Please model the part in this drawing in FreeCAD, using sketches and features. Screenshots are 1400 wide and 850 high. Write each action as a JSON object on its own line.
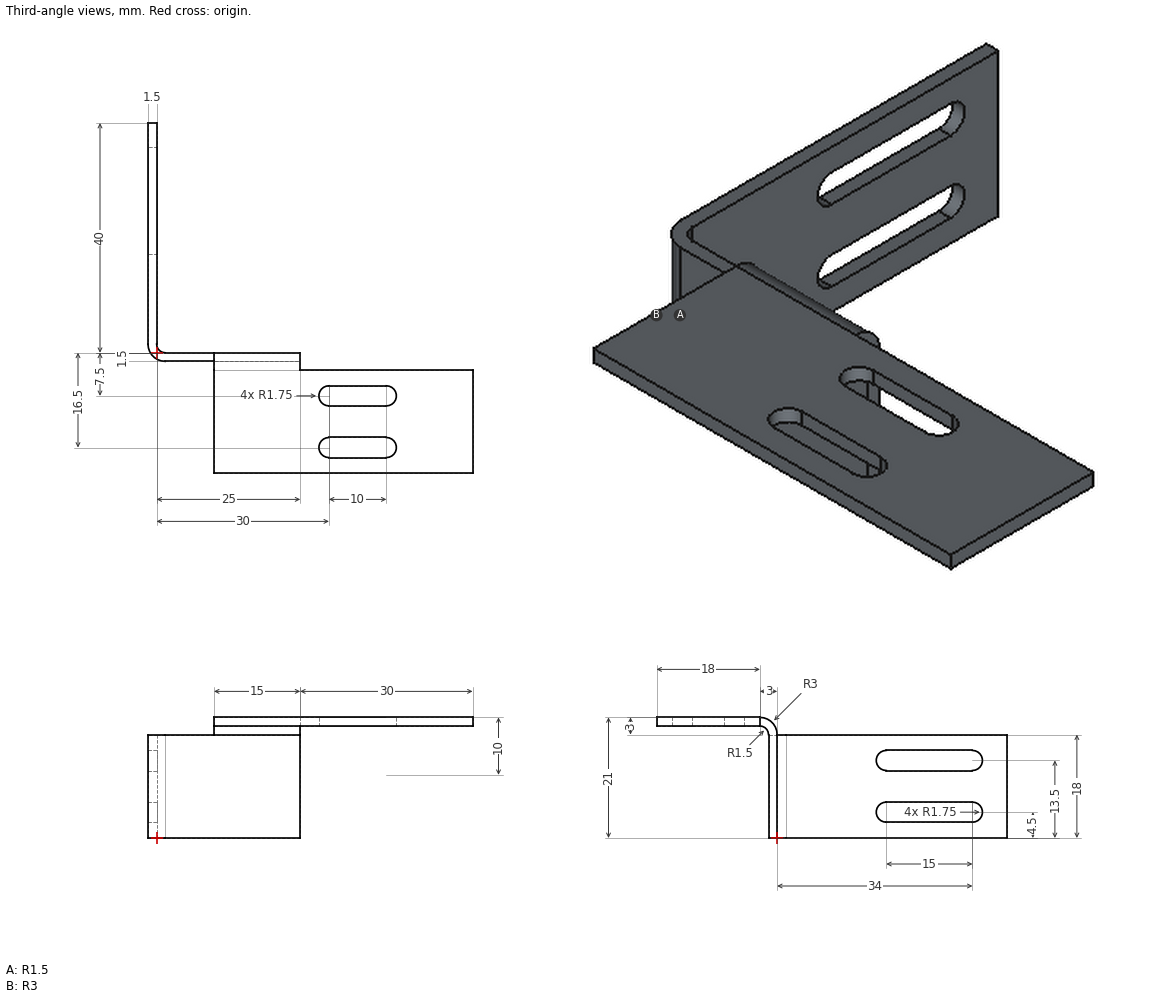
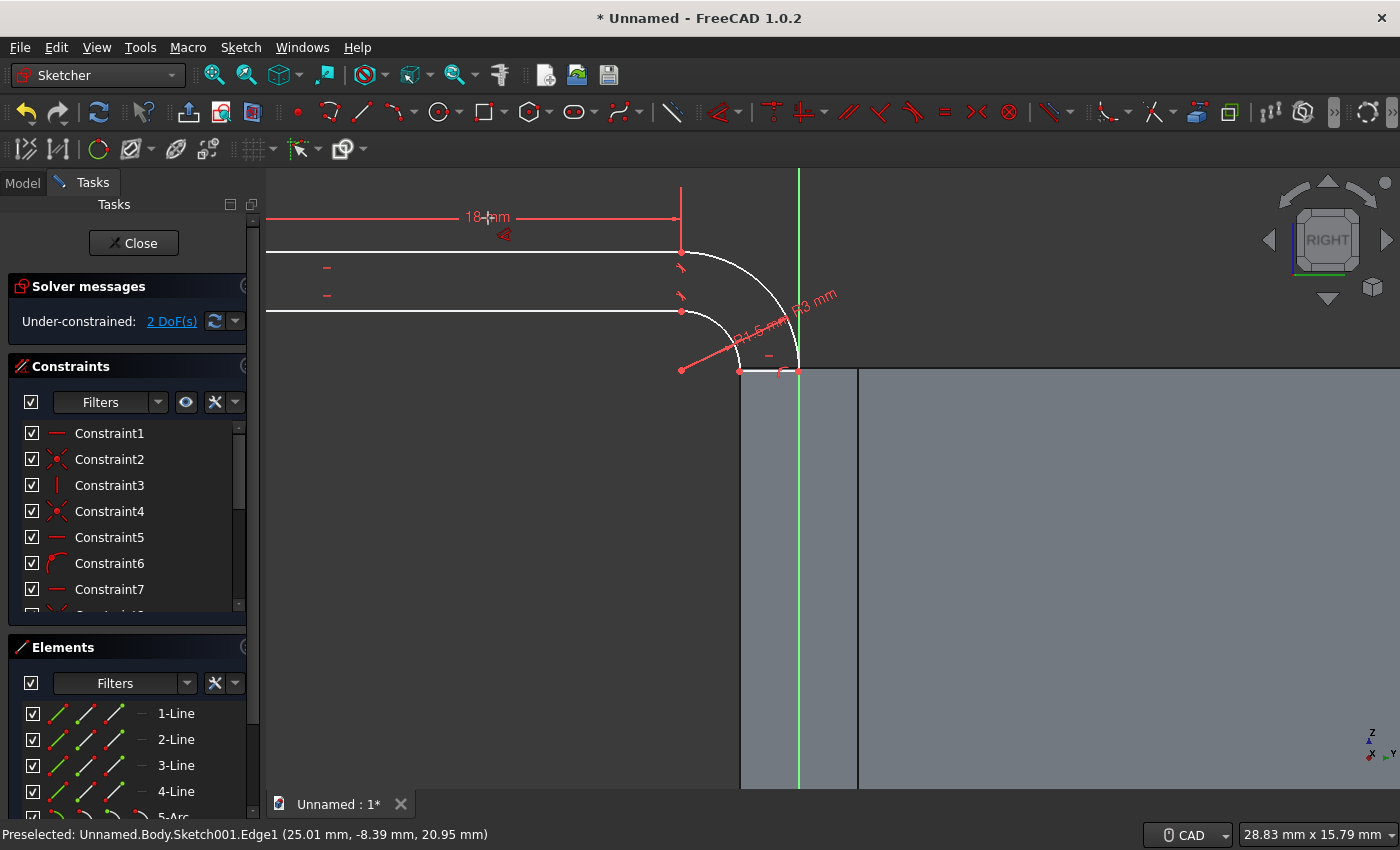
{"action": "left_click", "coordinate": [681, 252]}
{"action": "left_click", "coordinate": [833, 507]}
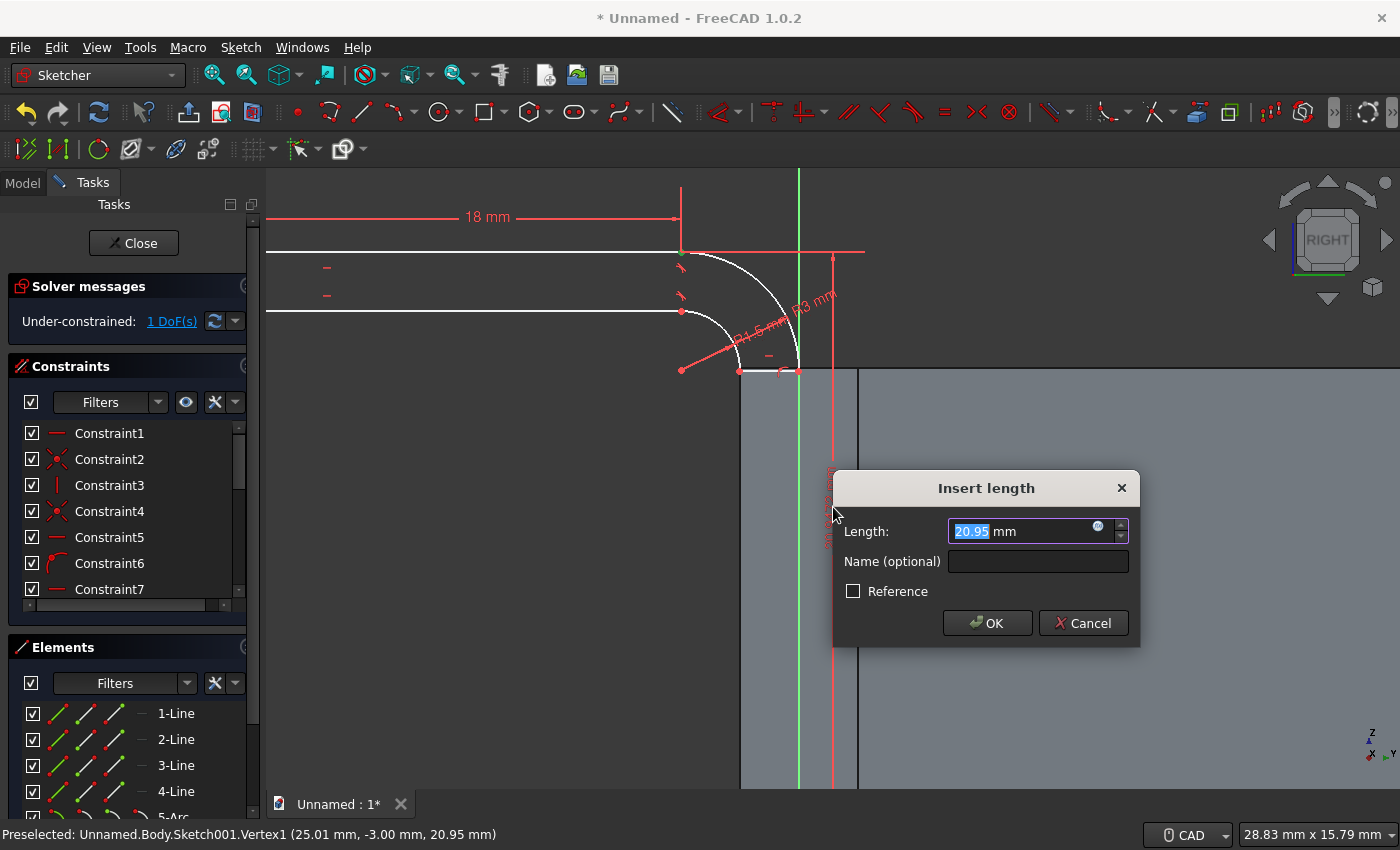
{"action": "type", "text": "21"}
{"action": "key", "text": "Return"}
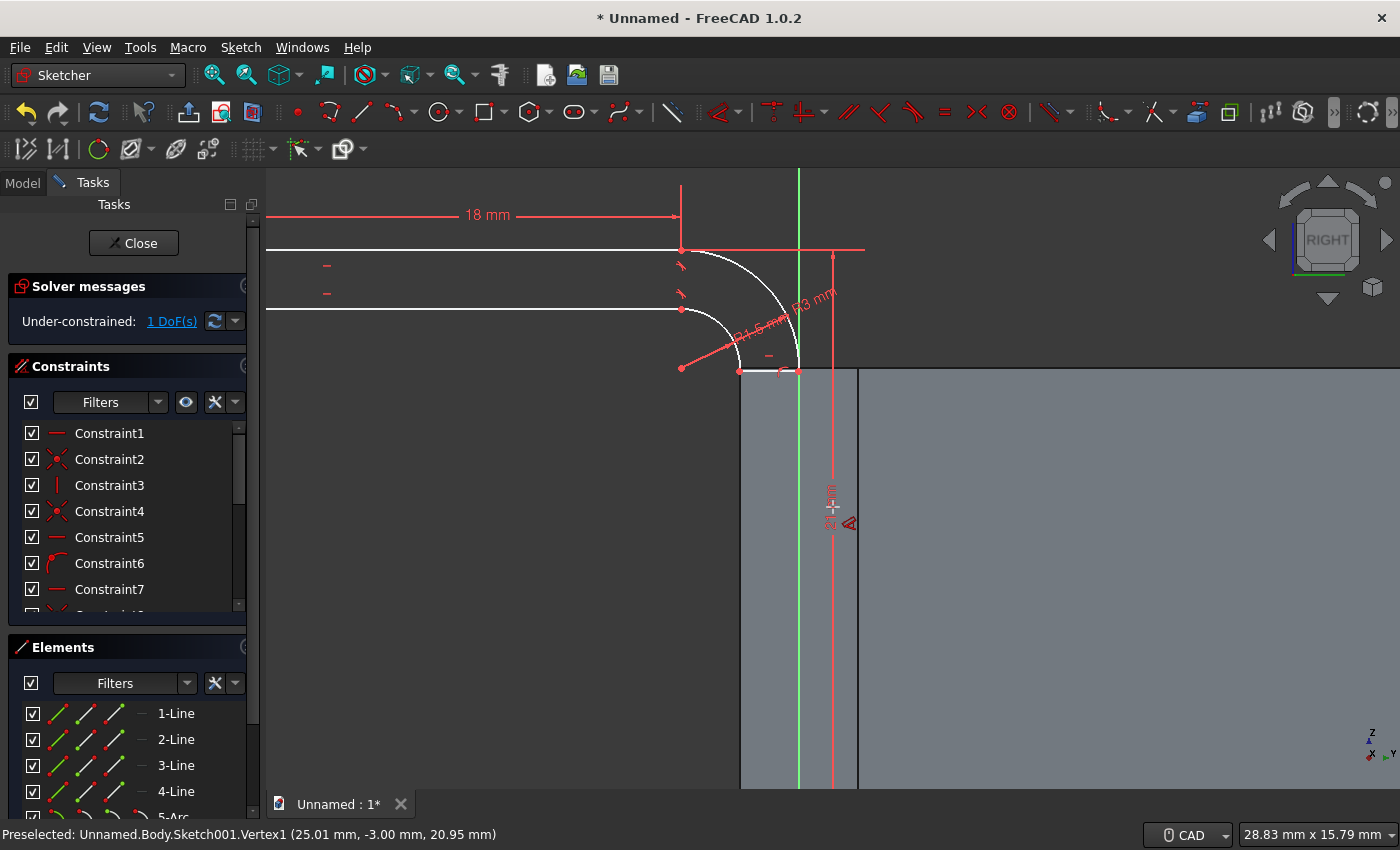
{"action": "left_click", "coordinate": [740, 371]}
{"action": "left_click", "coordinate": [833, 566]}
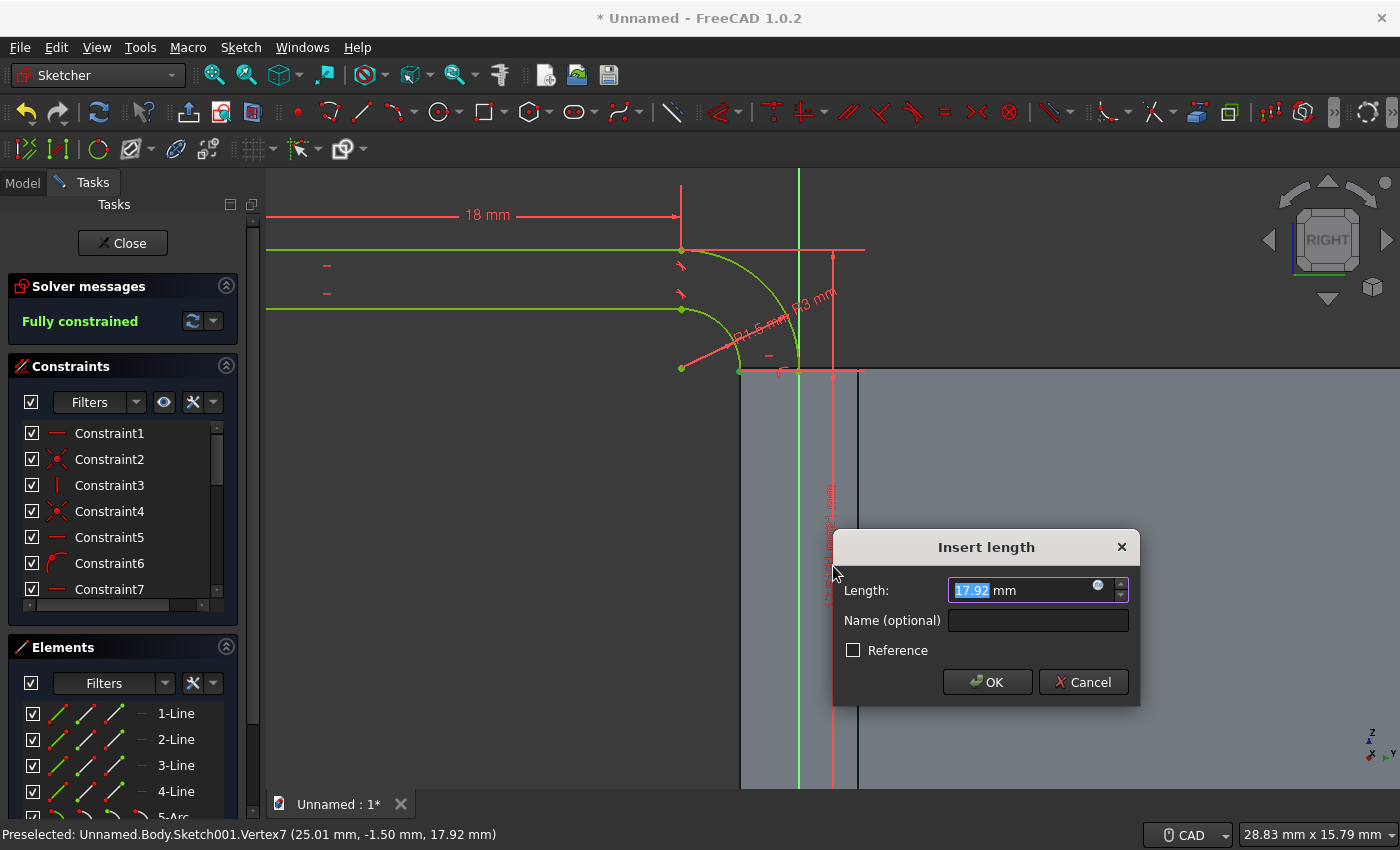
{"action": "type", "text": "18"}
{"action": "key", "text": "Return"}
{"action": "key", "text": "Escape"}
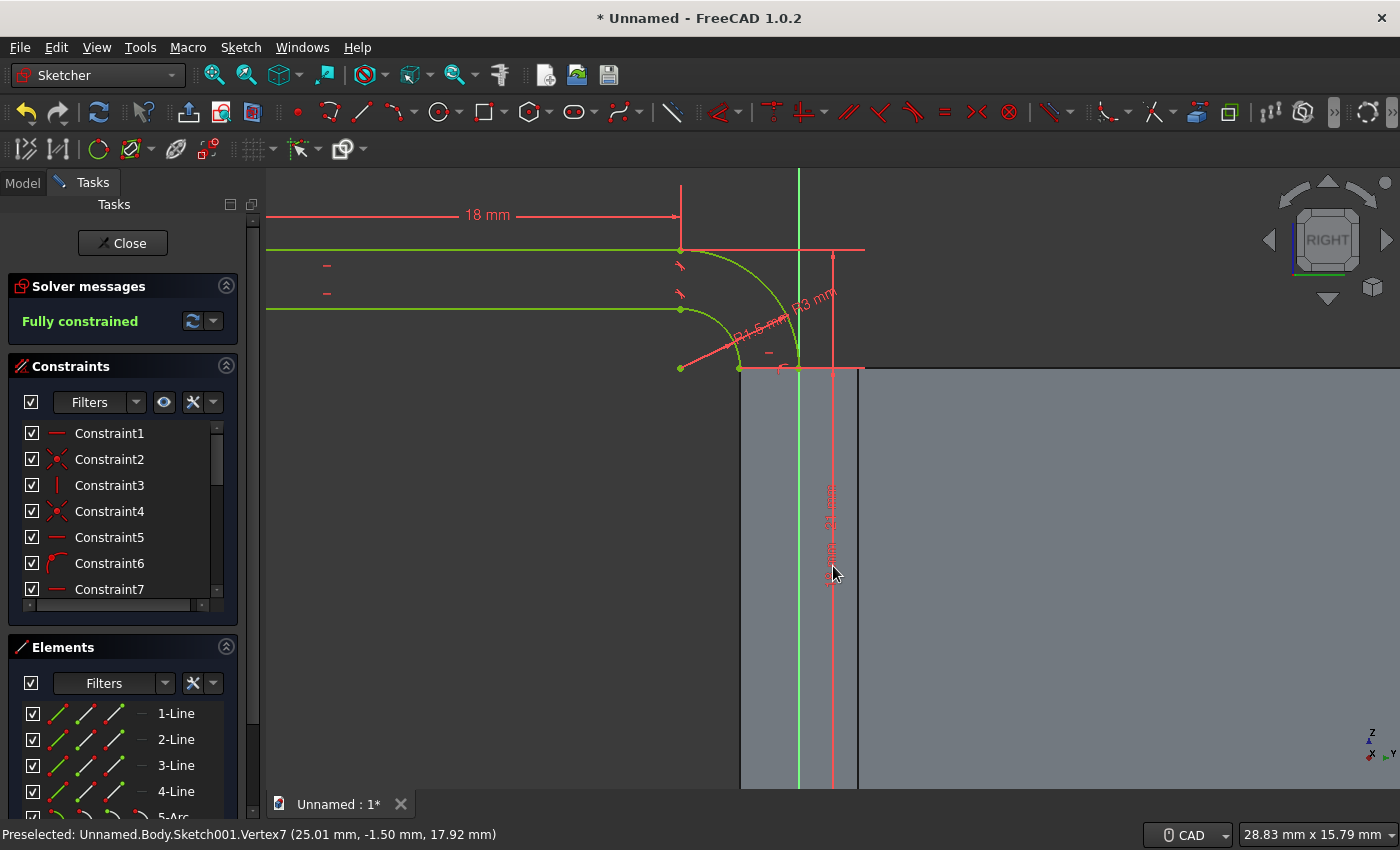
{"action": "left_click", "coordinate": [123, 243]}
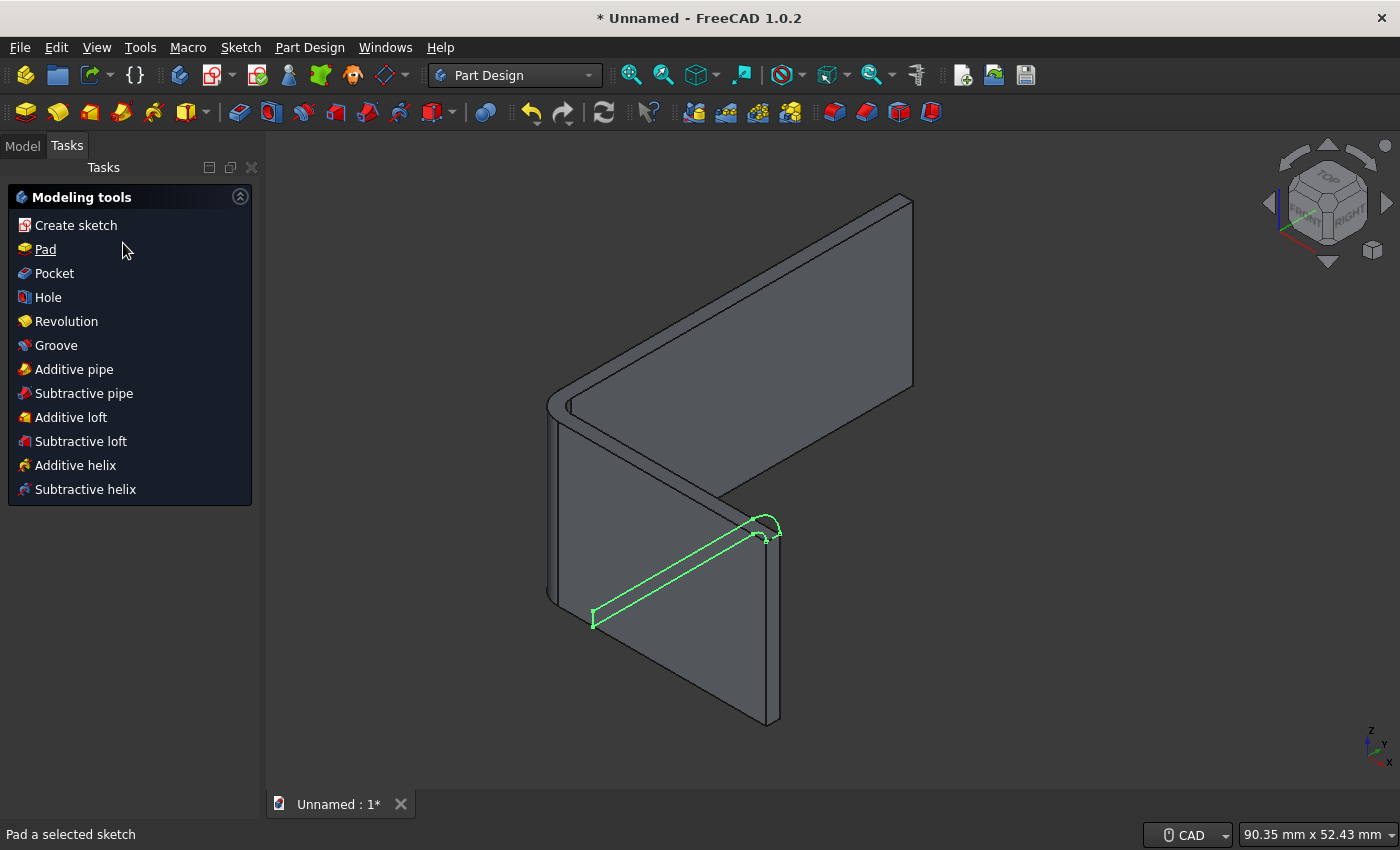
{"action": "left_click", "coordinate": [26, 112]}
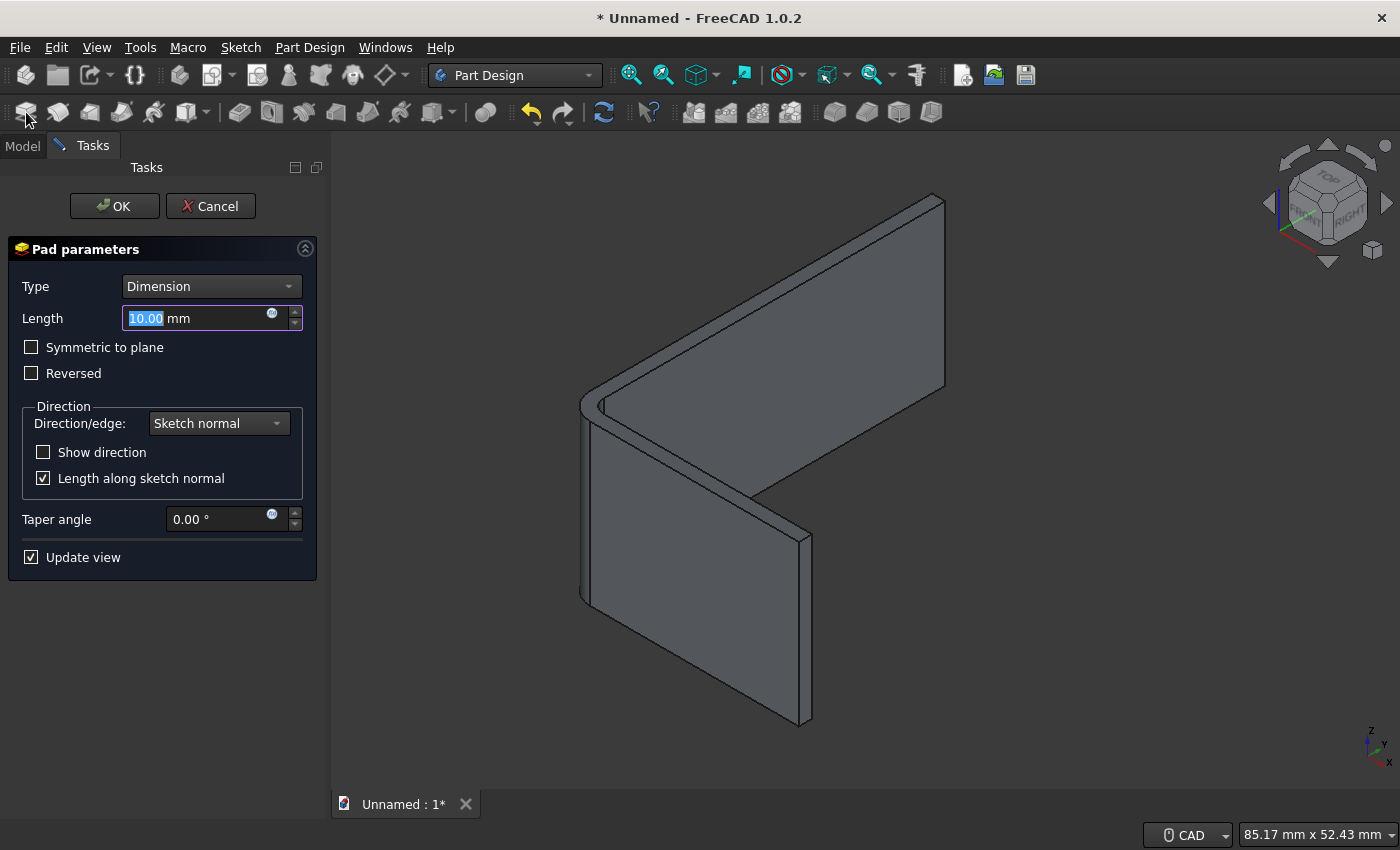
{"action": "left_click", "coordinate": [212, 286]}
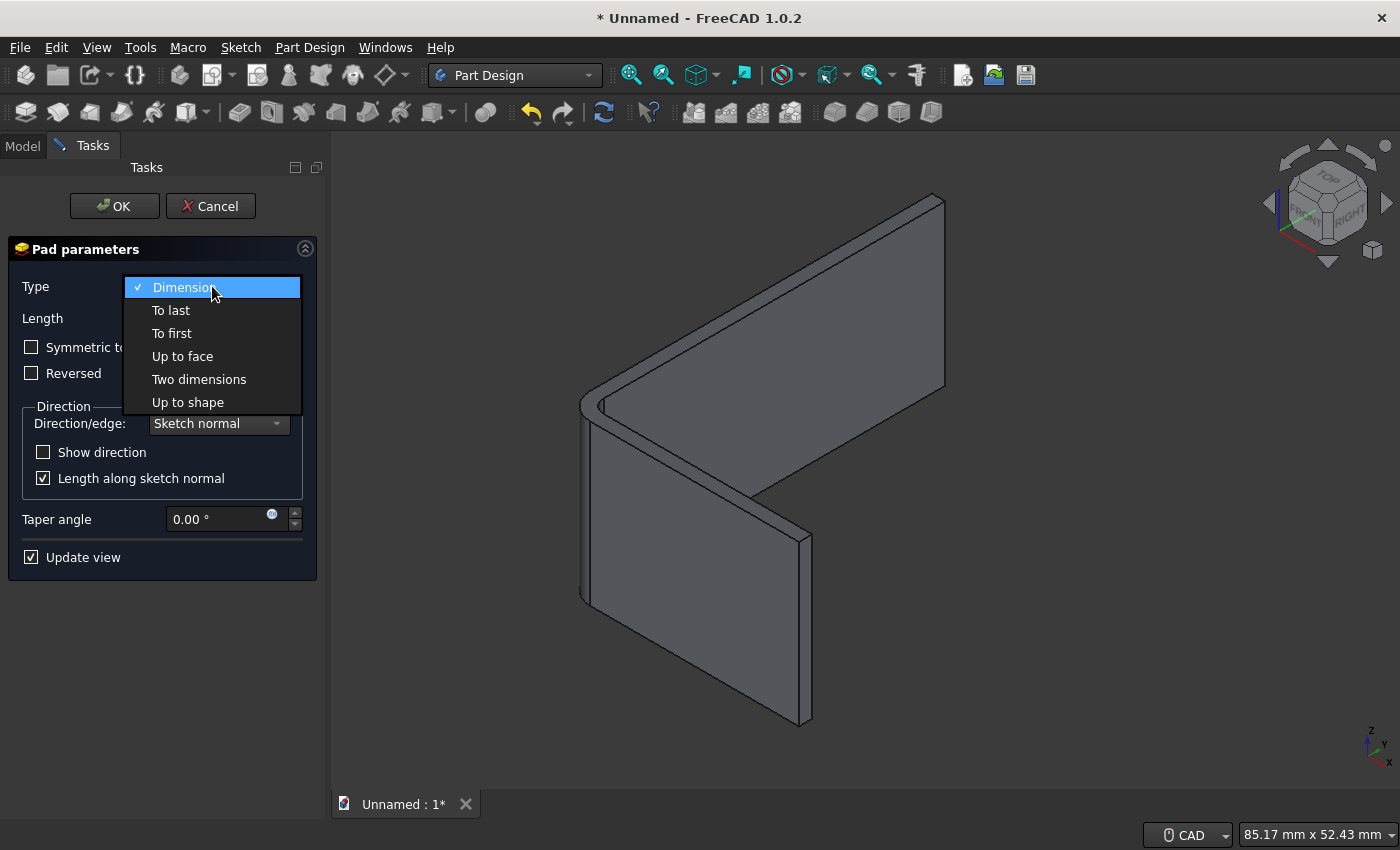
{"action": "left_click", "coordinate": [212, 380]}